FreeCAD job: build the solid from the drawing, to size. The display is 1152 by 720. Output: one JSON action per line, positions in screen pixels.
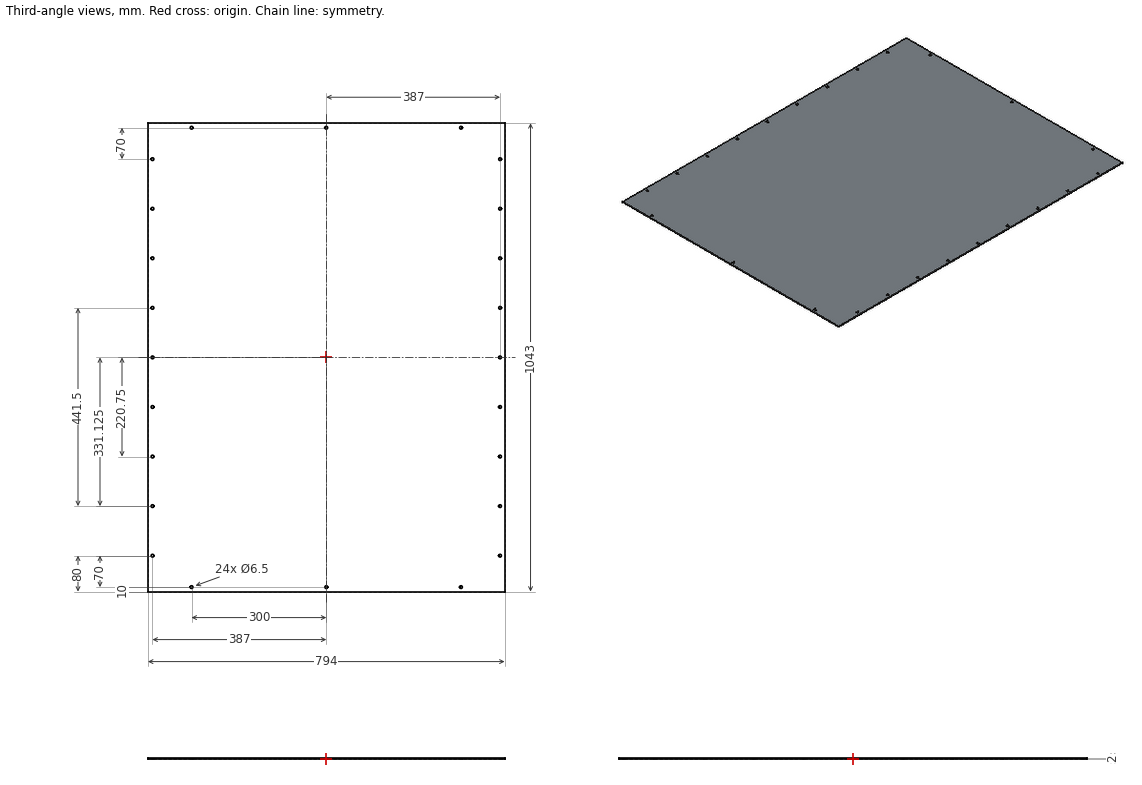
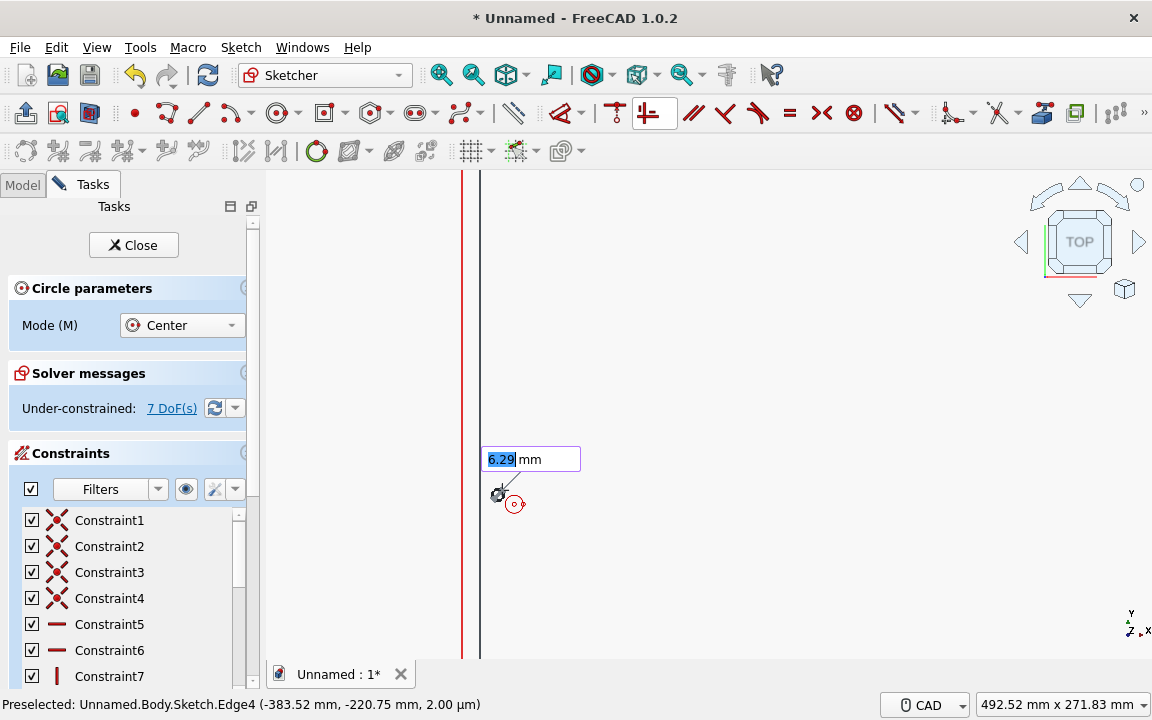
{"action": "type", "text": "6.5"}
{"action": "key", "text": "Return"}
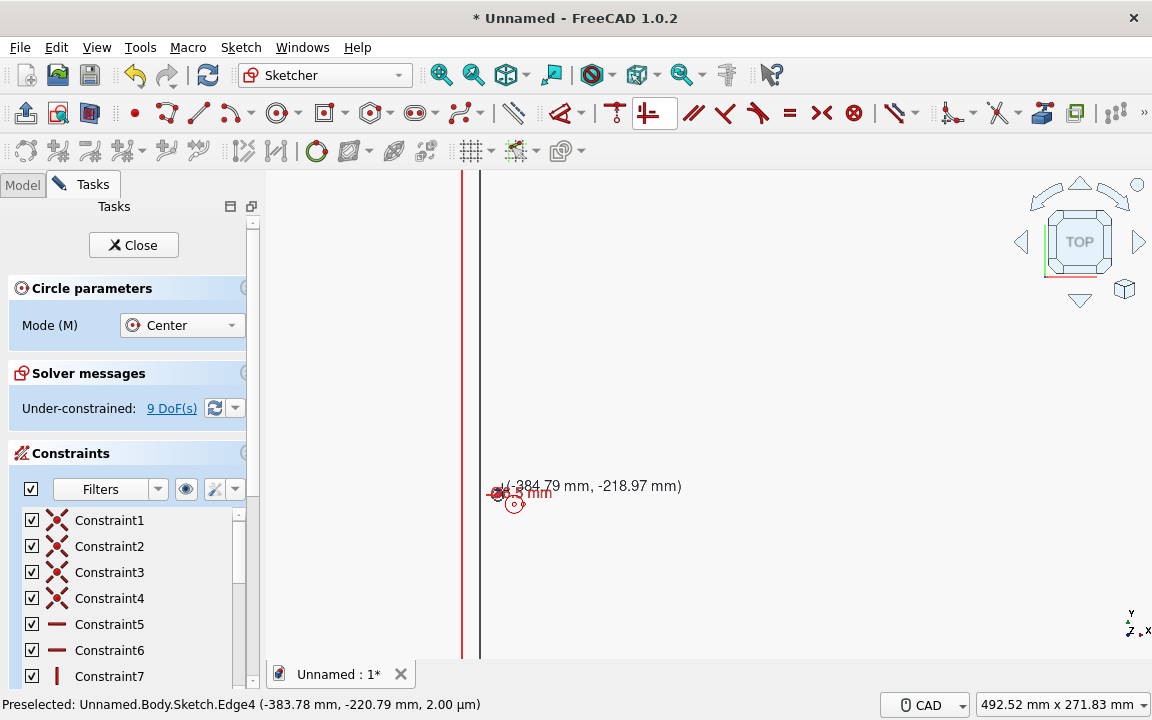
{"action": "scroll", "coordinate": [498, 296], "scroll_direction": "up", "scroll_amount": 7}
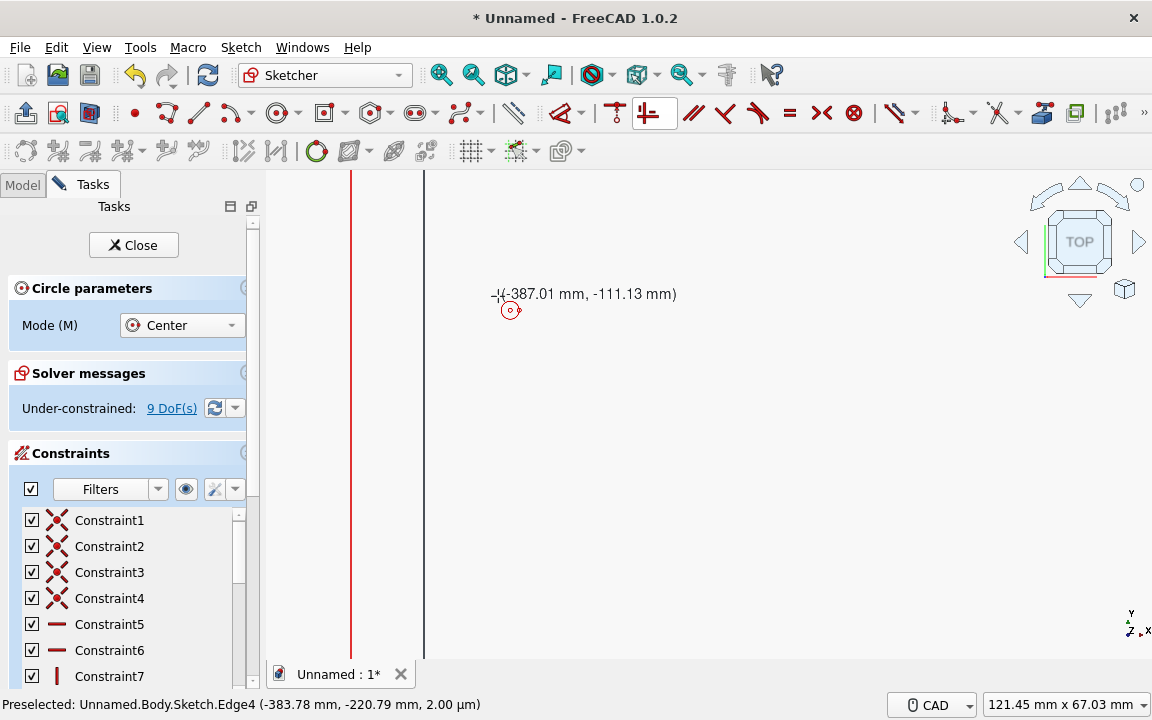
{"action": "scroll", "coordinate": [500, 463], "scroll_direction": "down", "scroll_amount": 15}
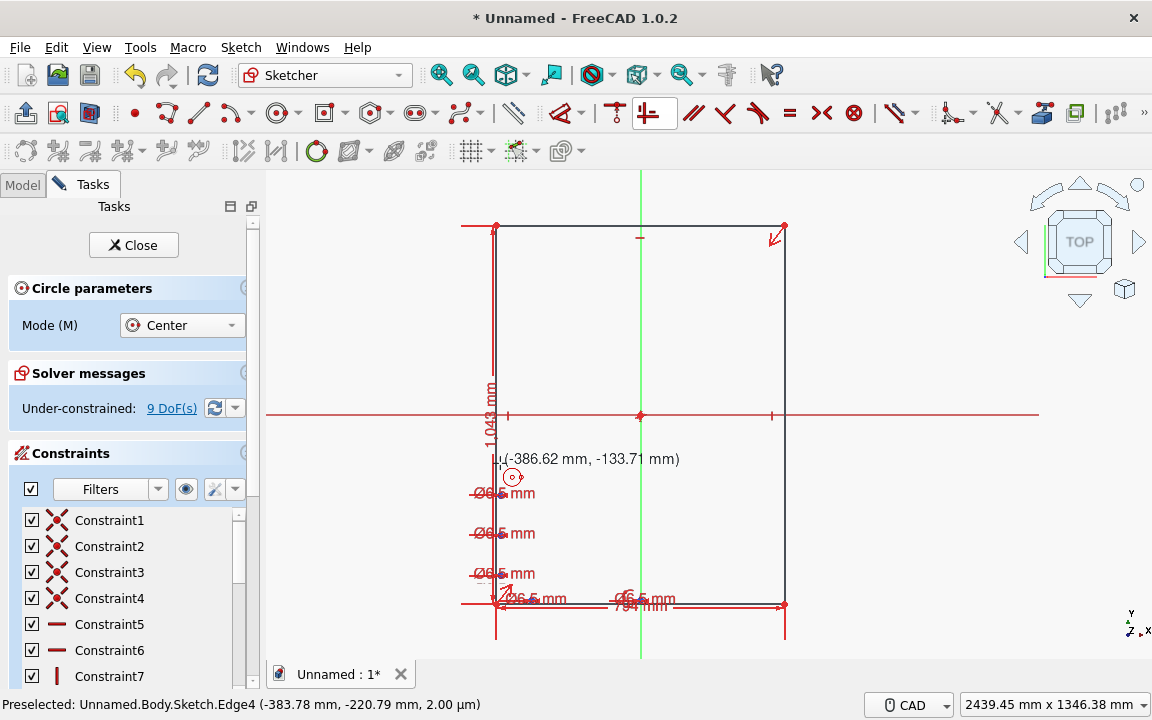
{"action": "scroll", "coordinate": [500, 455], "scroll_direction": "up", "scroll_amount": 8}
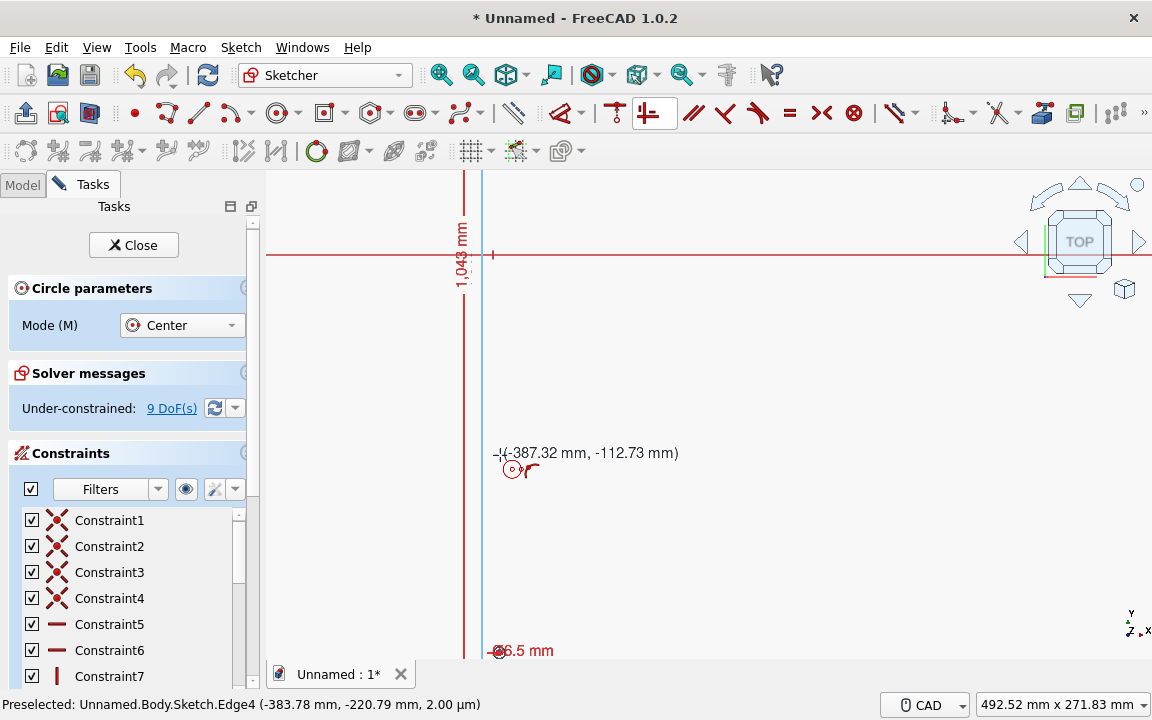
{"action": "left_click", "coordinate": [500, 453]}
{"action": "mouse_move", "coordinate": [504, 449]}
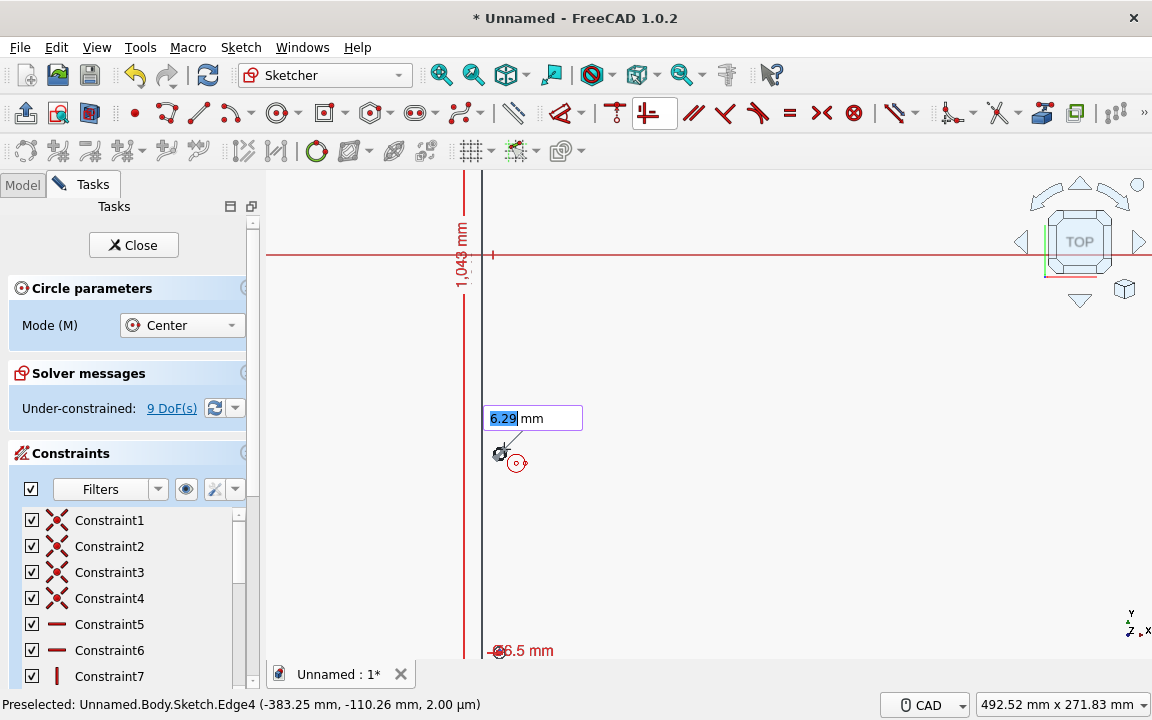
{"action": "type", "text": "6.5"}
{"action": "key", "text": "Return"}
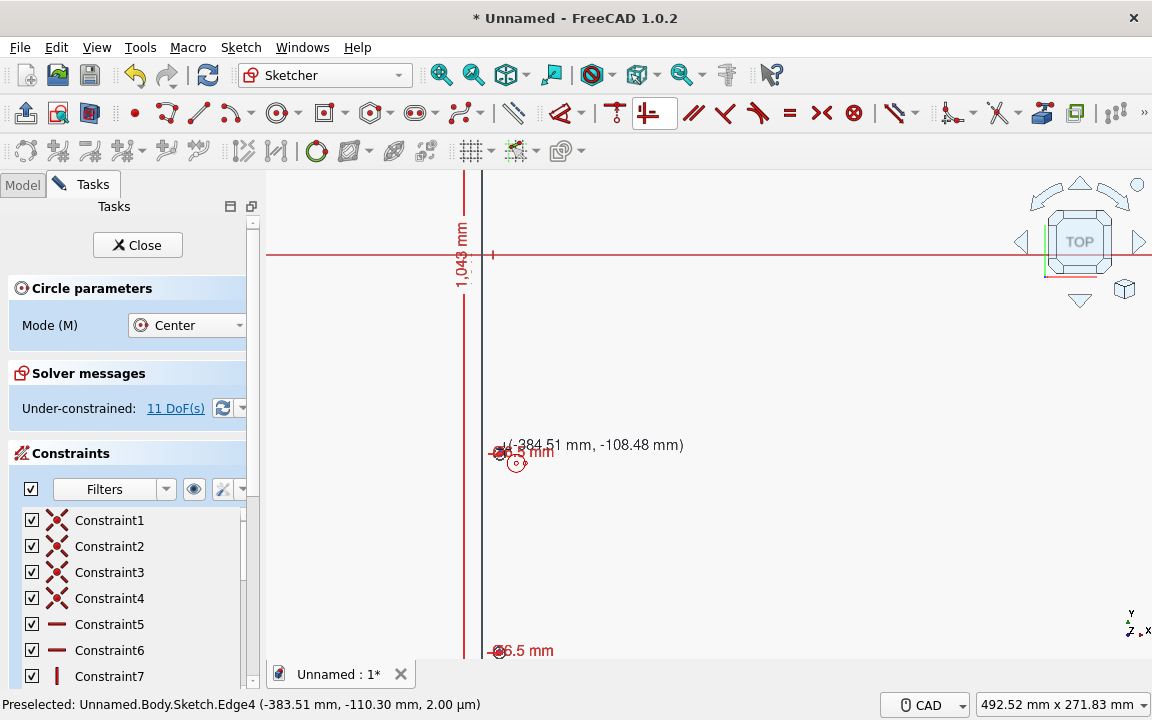
{"action": "scroll", "coordinate": [531, 446], "scroll_direction": "down", "scroll_amount": 9}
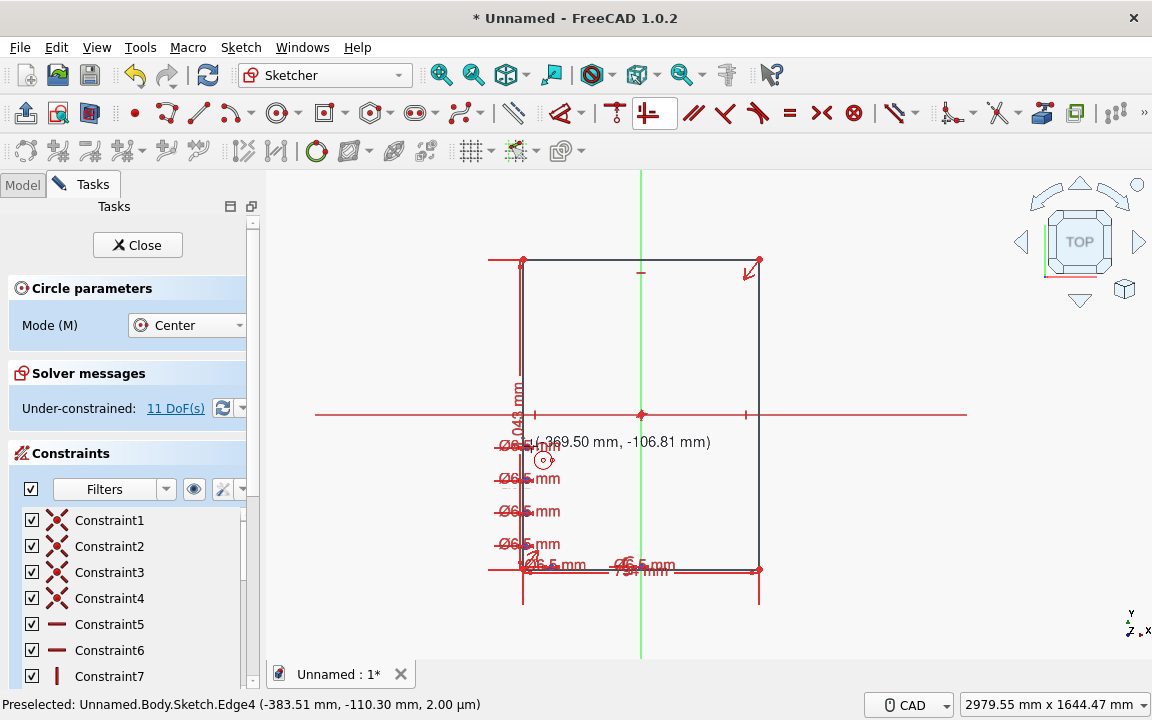
{"action": "scroll", "coordinate": [730, 567], "scroll_direction": "up", "scroll_amount": 16}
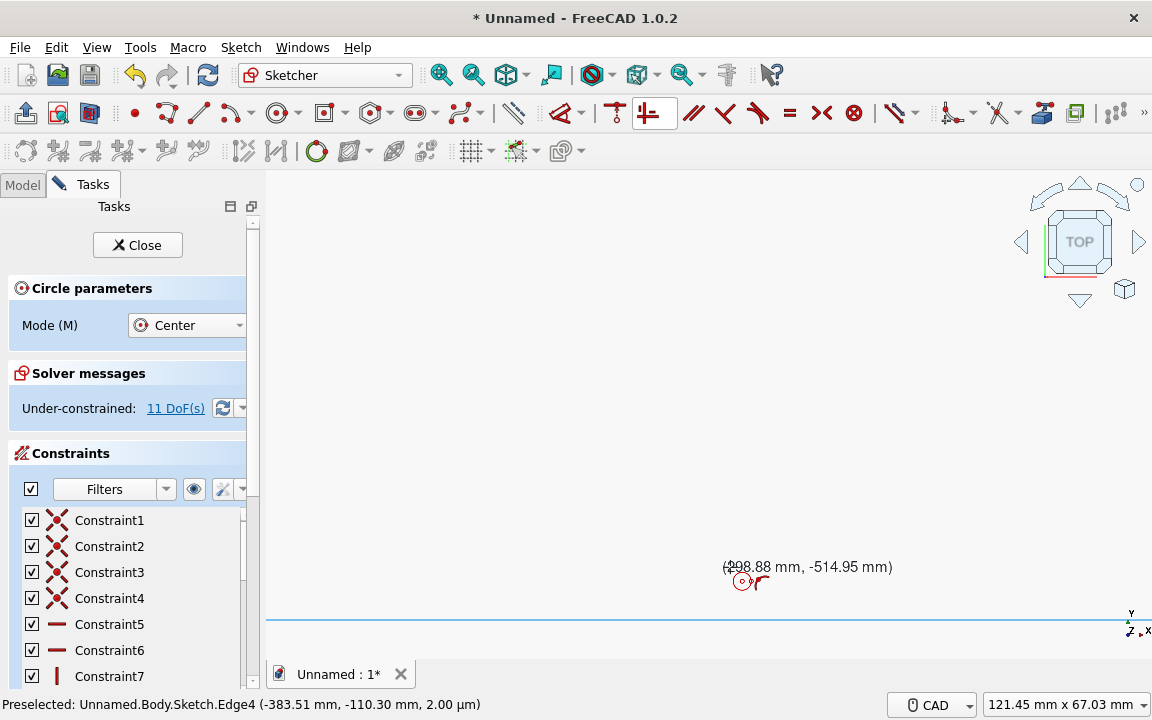
{"action": "scroll", "coordinate": [751, 603], "scroll_direction": "down", "scroll_amount": 15}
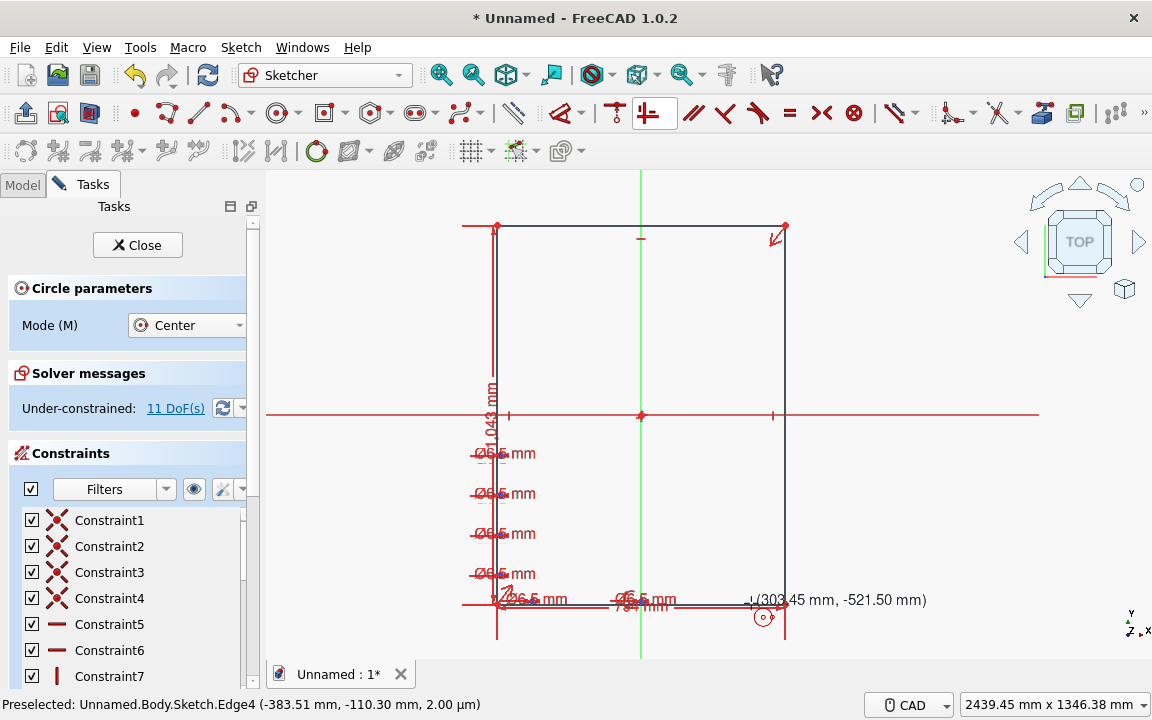
{"action": "scroll", "coordinate": [750, 601], "scroll_direction": "up", "scroll_amount": 8}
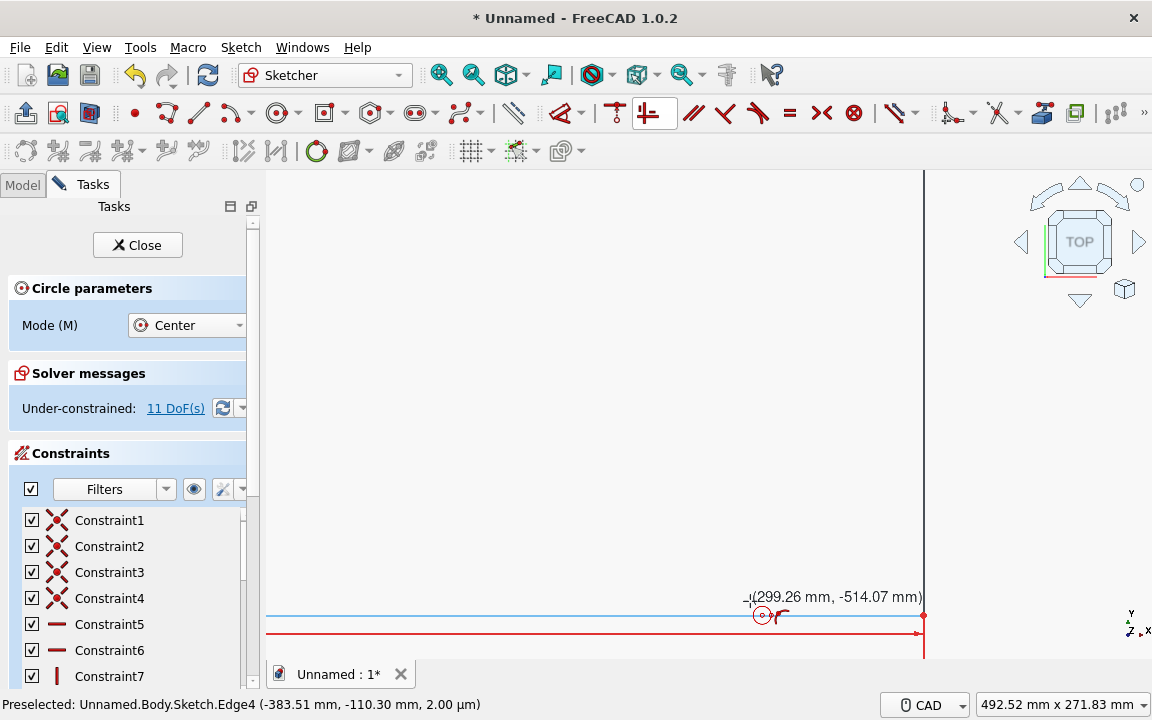
{"action": "left_click", "coordinate": [749, 598]}
{"action": "mouse_move", "coordinate": [753, 594]}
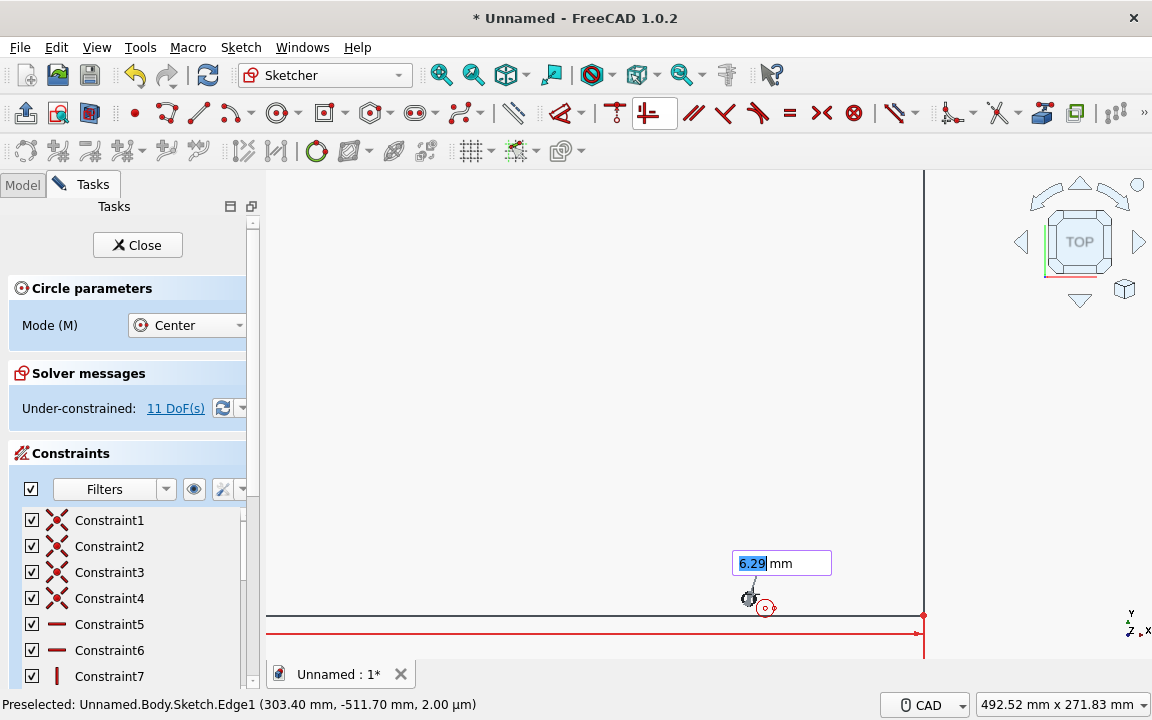
{"action": "type", "text": "6.5"}
{"action": "key", "text": "Return"}